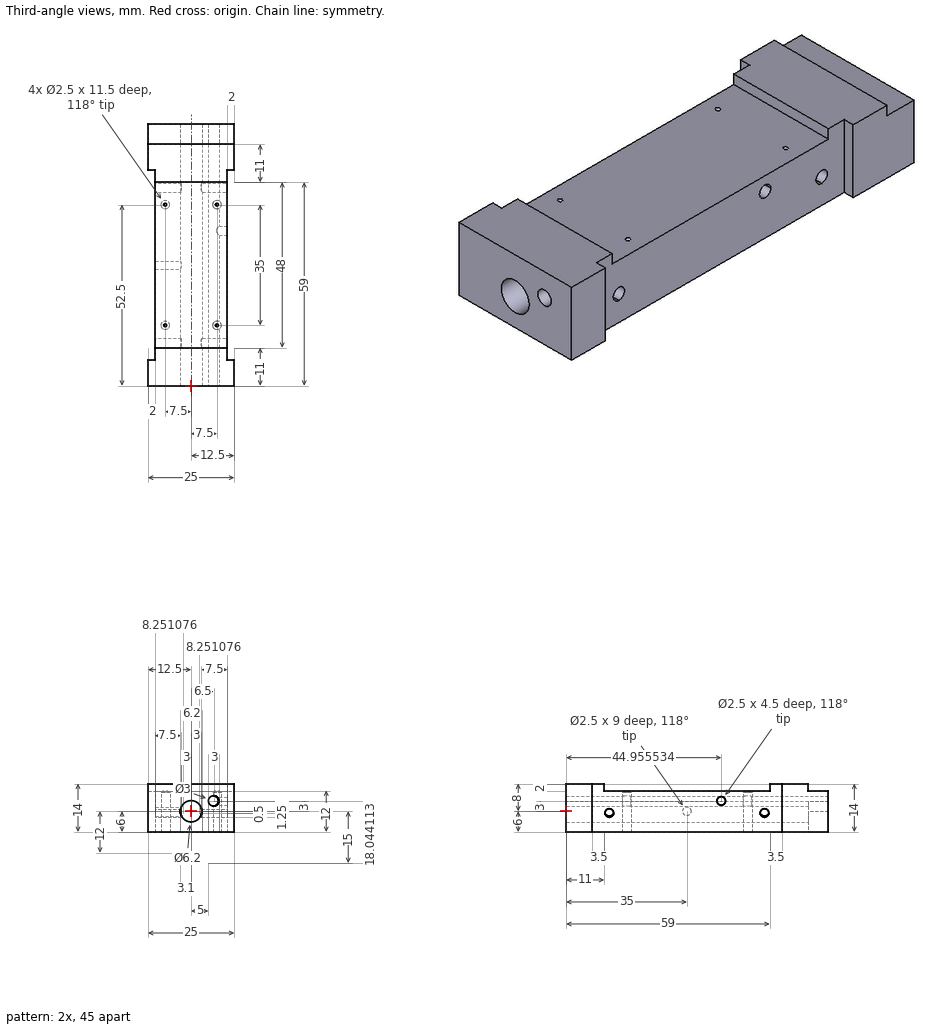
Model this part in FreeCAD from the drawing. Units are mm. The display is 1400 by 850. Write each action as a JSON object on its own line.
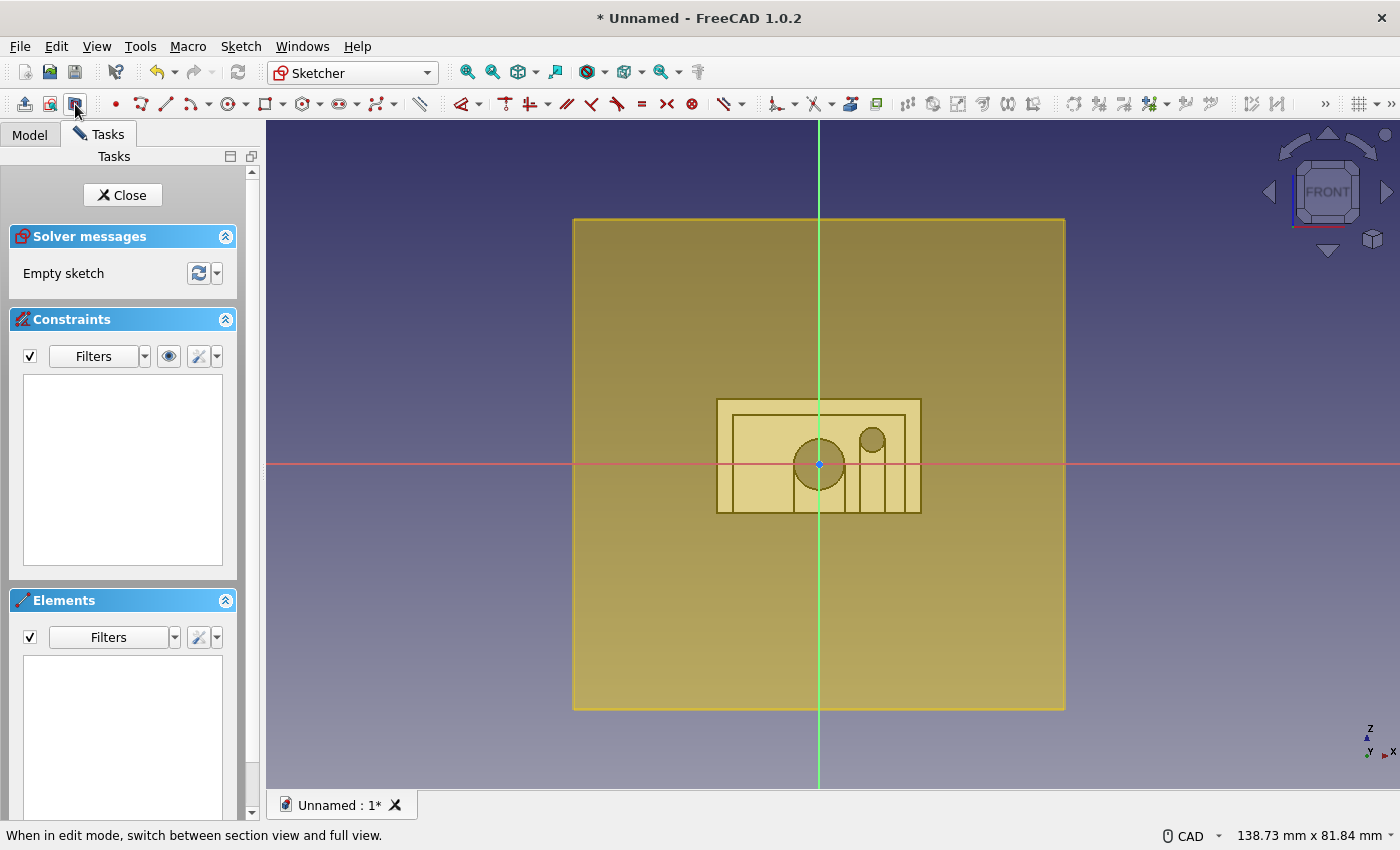
{"action": "scroll", "coordinate": [872, 474], "scroll_direction": "up", "scroll_amount": 10}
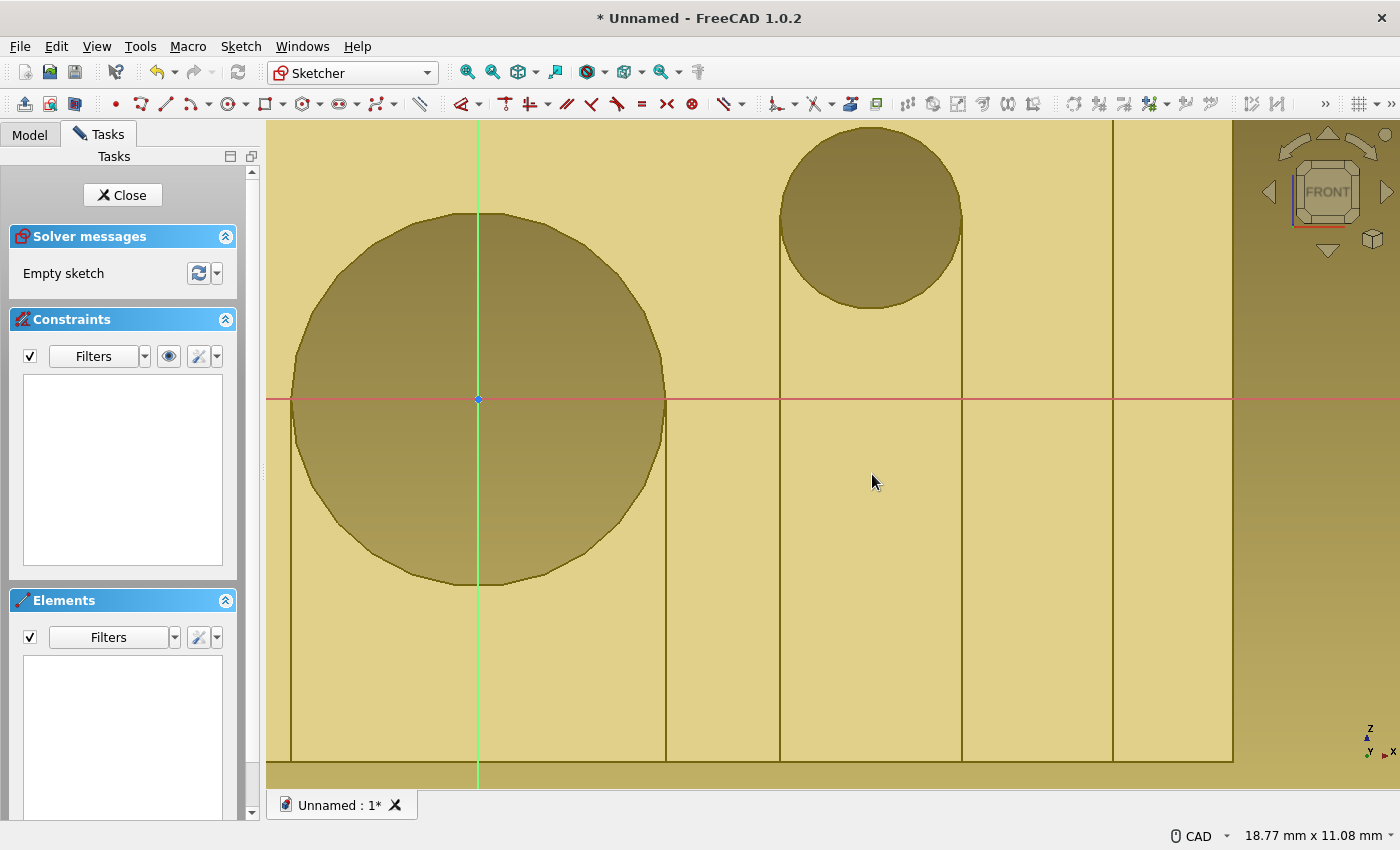
{"action": "left_click", "coordinate": [141, 104]}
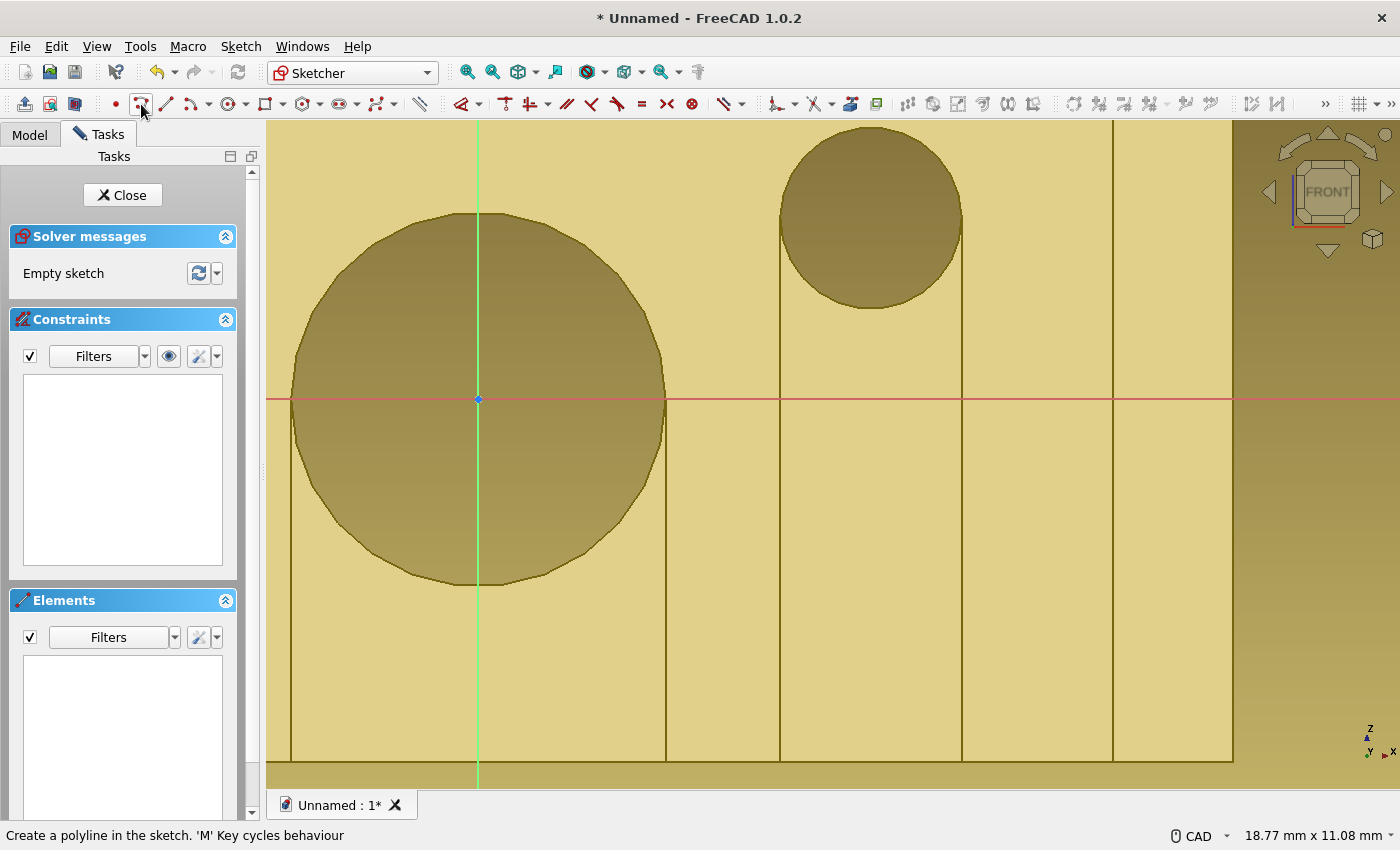
{"action": "left_click", "coordinate": [614, 430]}
{"action": "left_click", "coordinate": [1113, 430]}
{"action": "left_click", "coordinate": [1113, 505]}
{"action": "left_click", "coordinate": [660, 505]}
{"action": "left_click", "coordinate": [614, 431]}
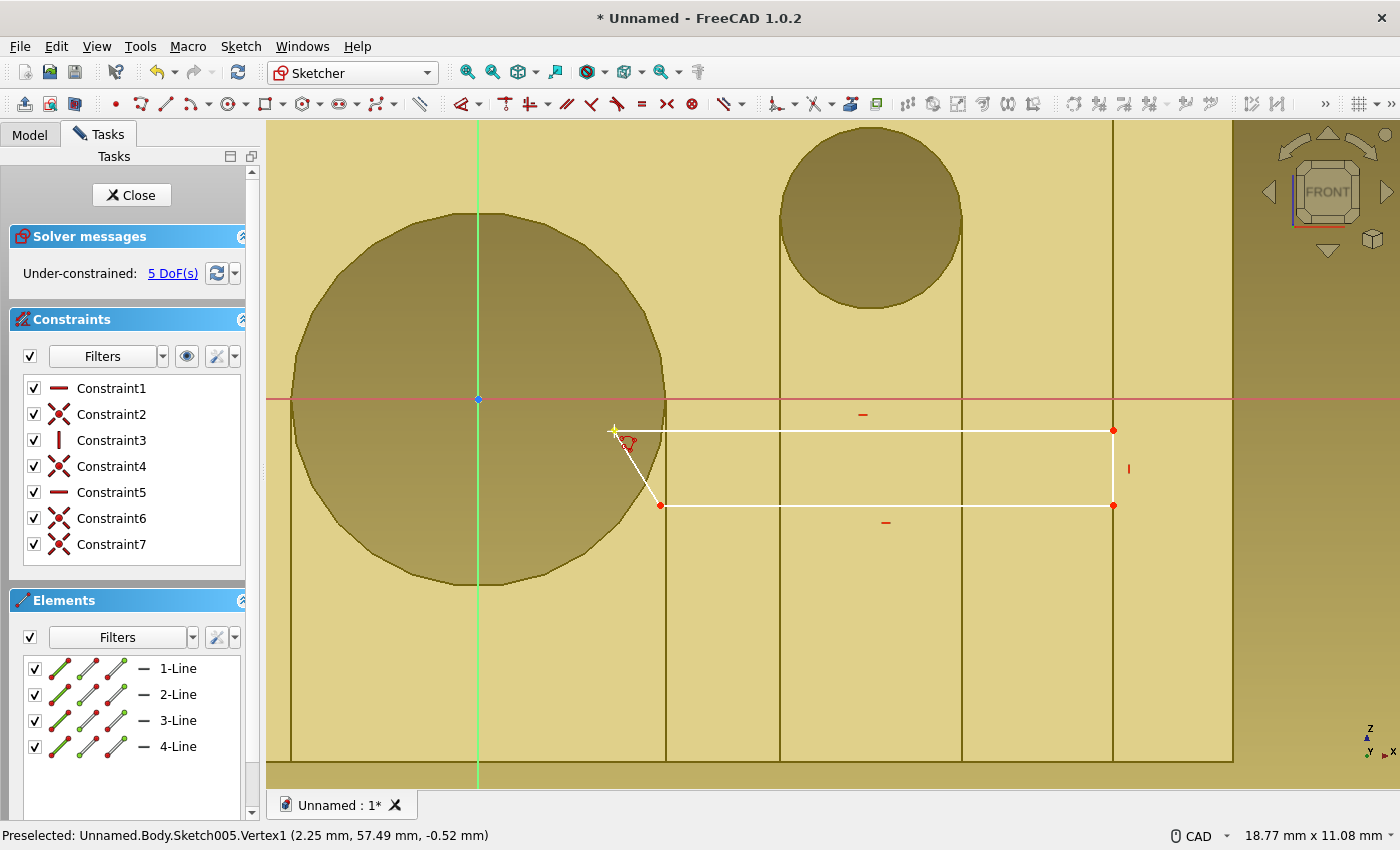
{"action": "left_click", "coordinate": [166, 104]}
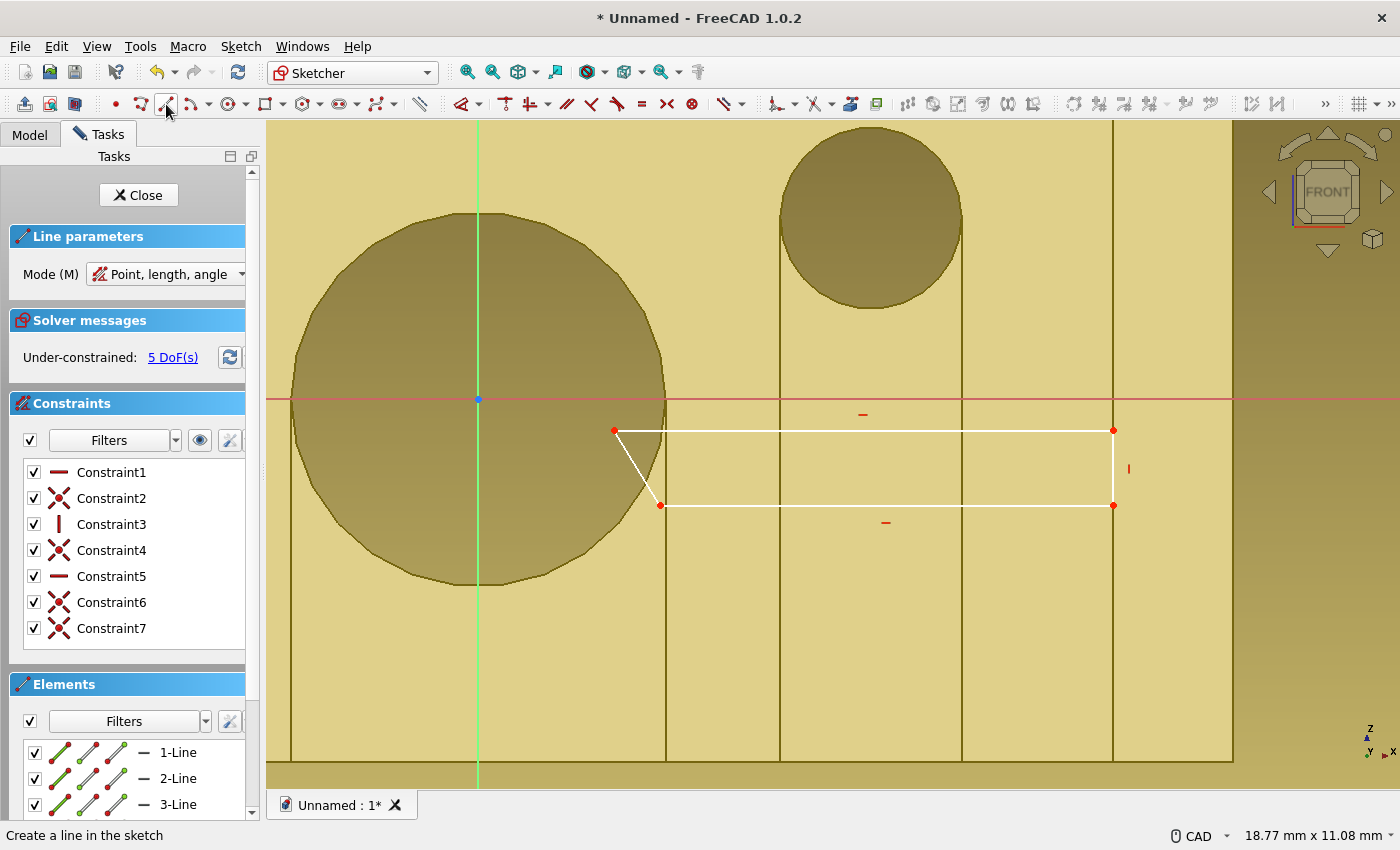
{"action": "left_click", "coordinate": [564, 430]}
{"action": "left_click", "coordinate": [415, 430]}
{"action": "key", "text": "Escape"}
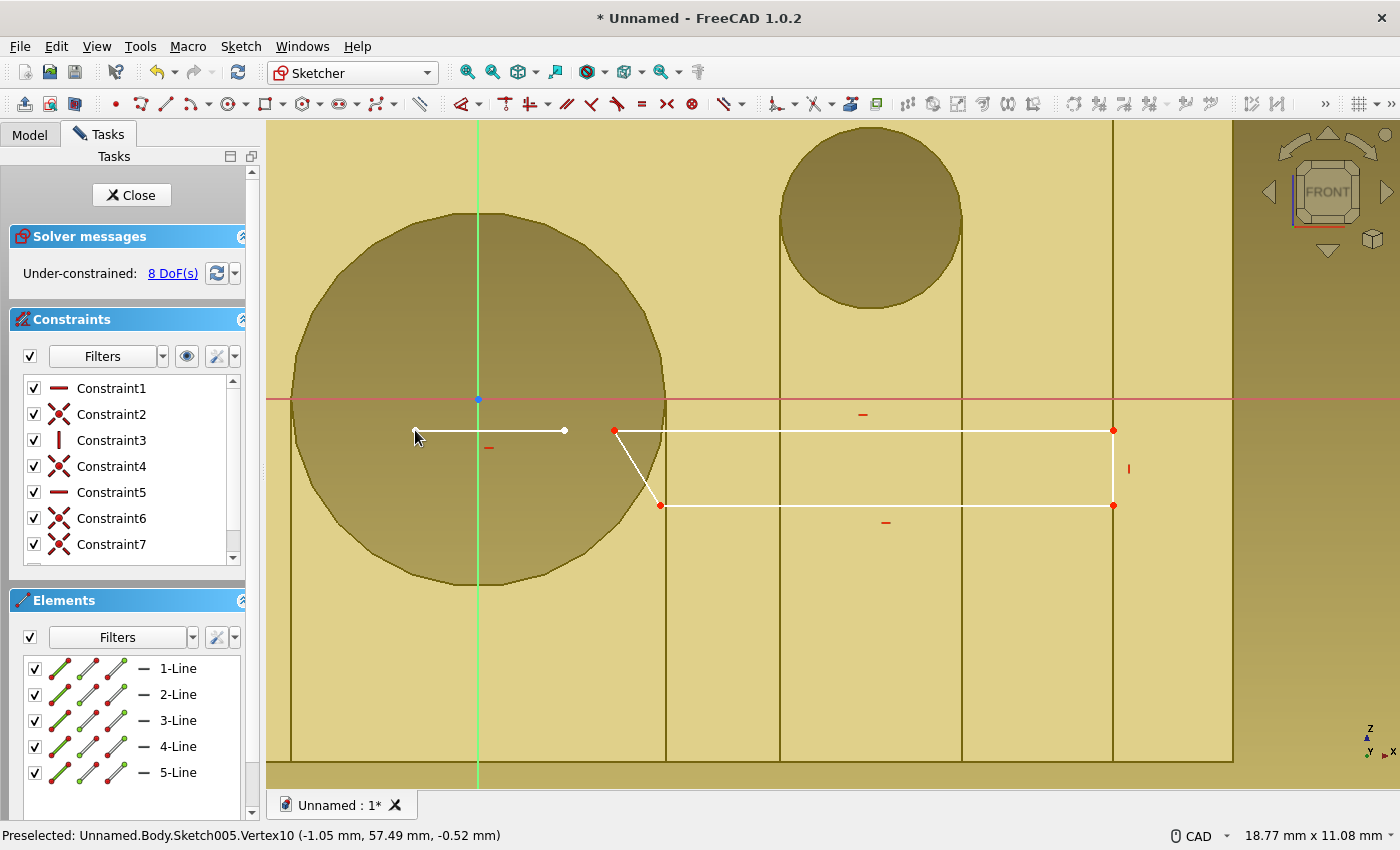
{"action": "left_click", "coordinate": [519, 431]}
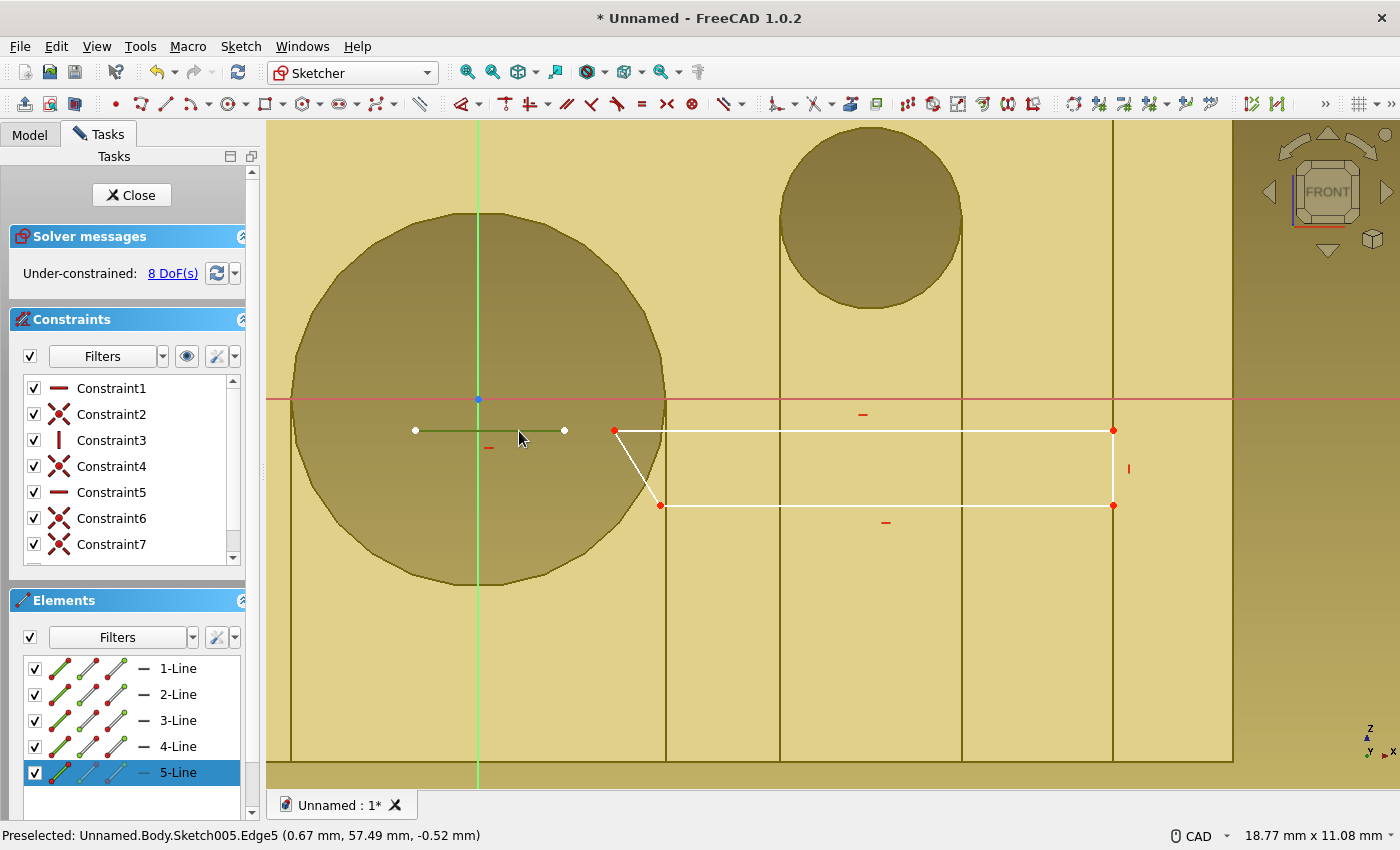
{"action": "left_click", "coordinate": [420, 104]}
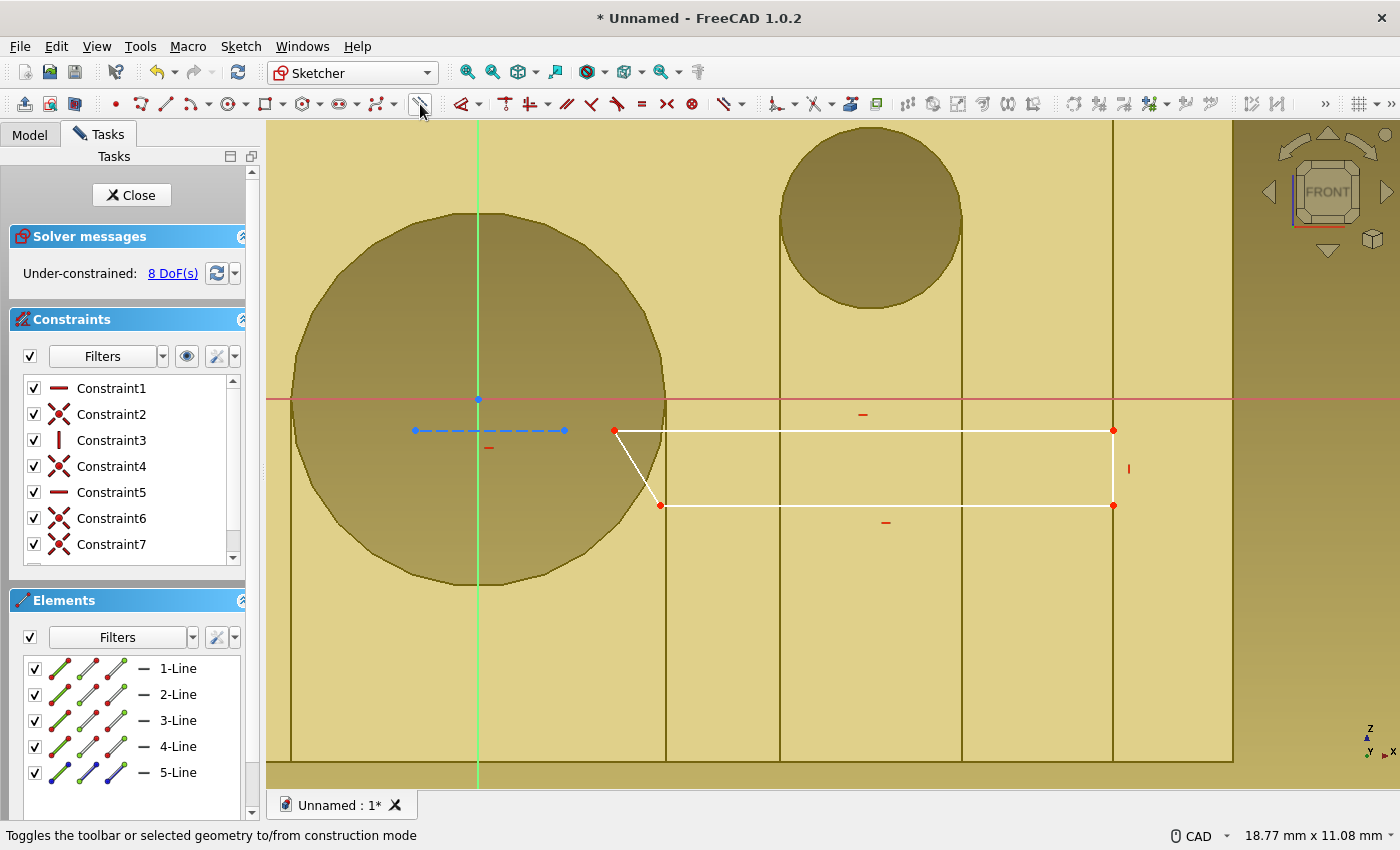
{"action": "left_click", "coordinate": [460, 104]}